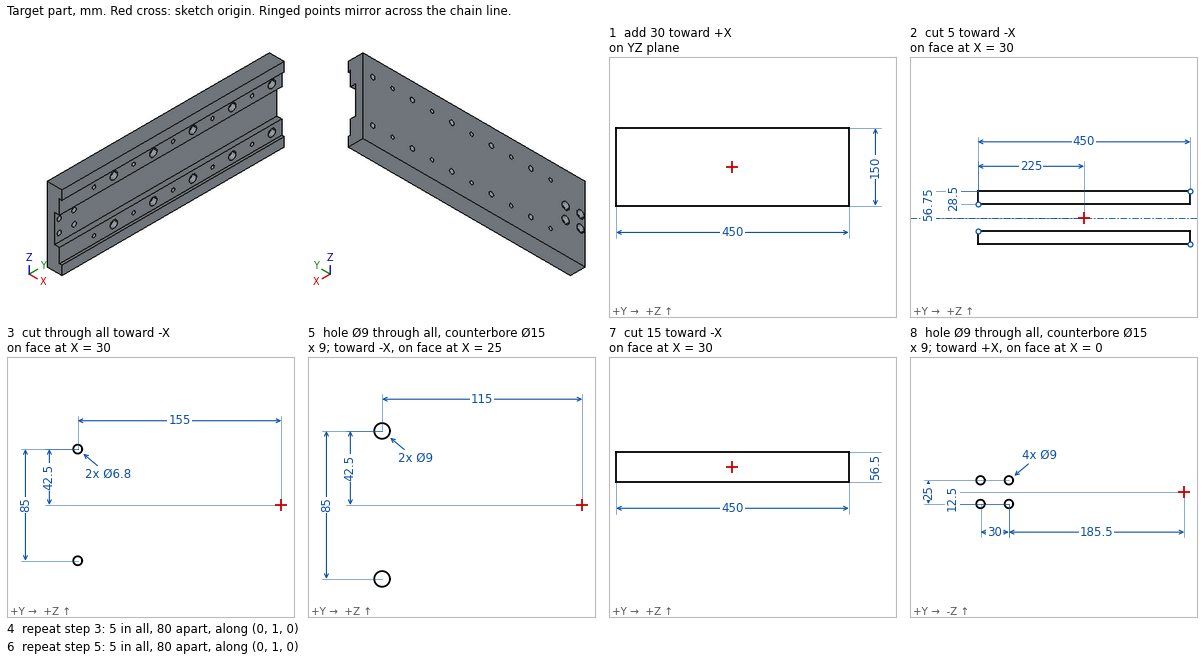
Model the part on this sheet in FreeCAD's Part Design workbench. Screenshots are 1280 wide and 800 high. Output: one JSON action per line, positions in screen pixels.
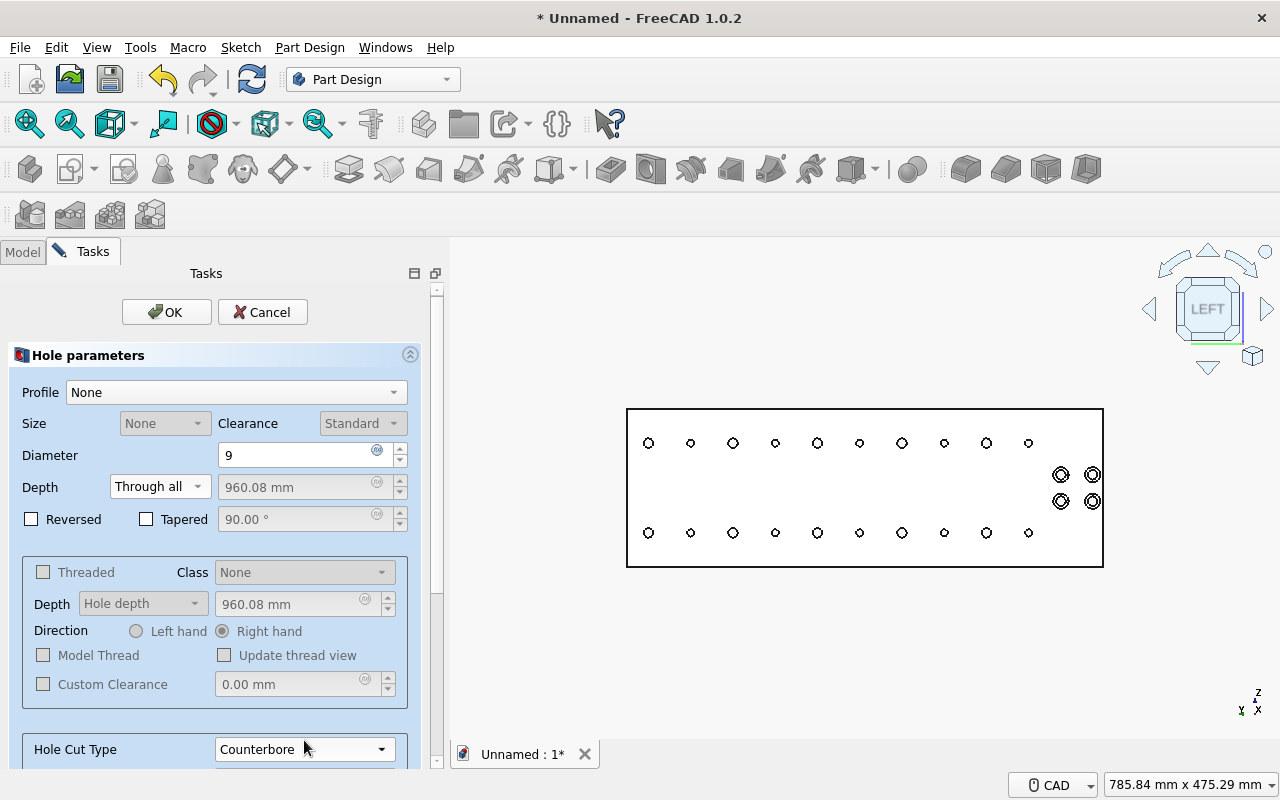
{"action": "scroll", "coordinate": [437, 526], "scroll_direction": "down", "scroll_amount": 2}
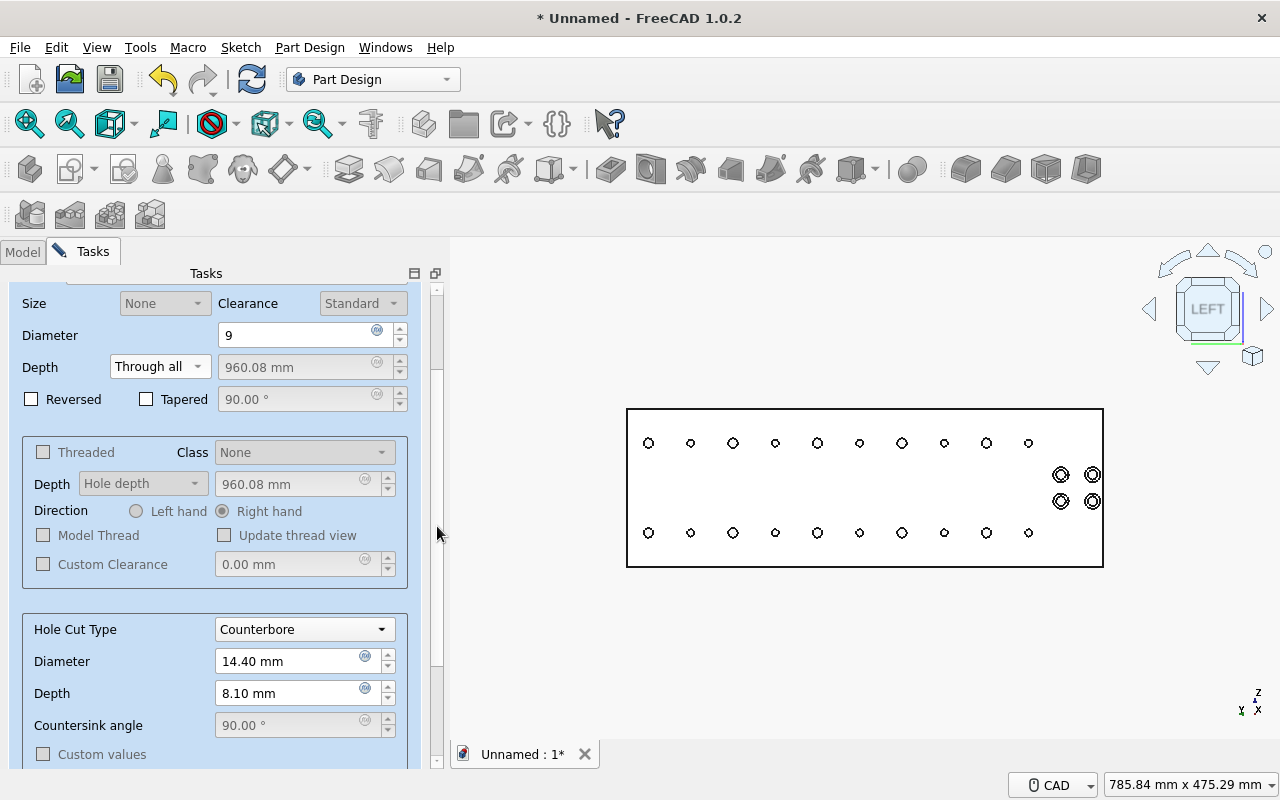
{"action": "triple_click", "coordinate": [298, 661]}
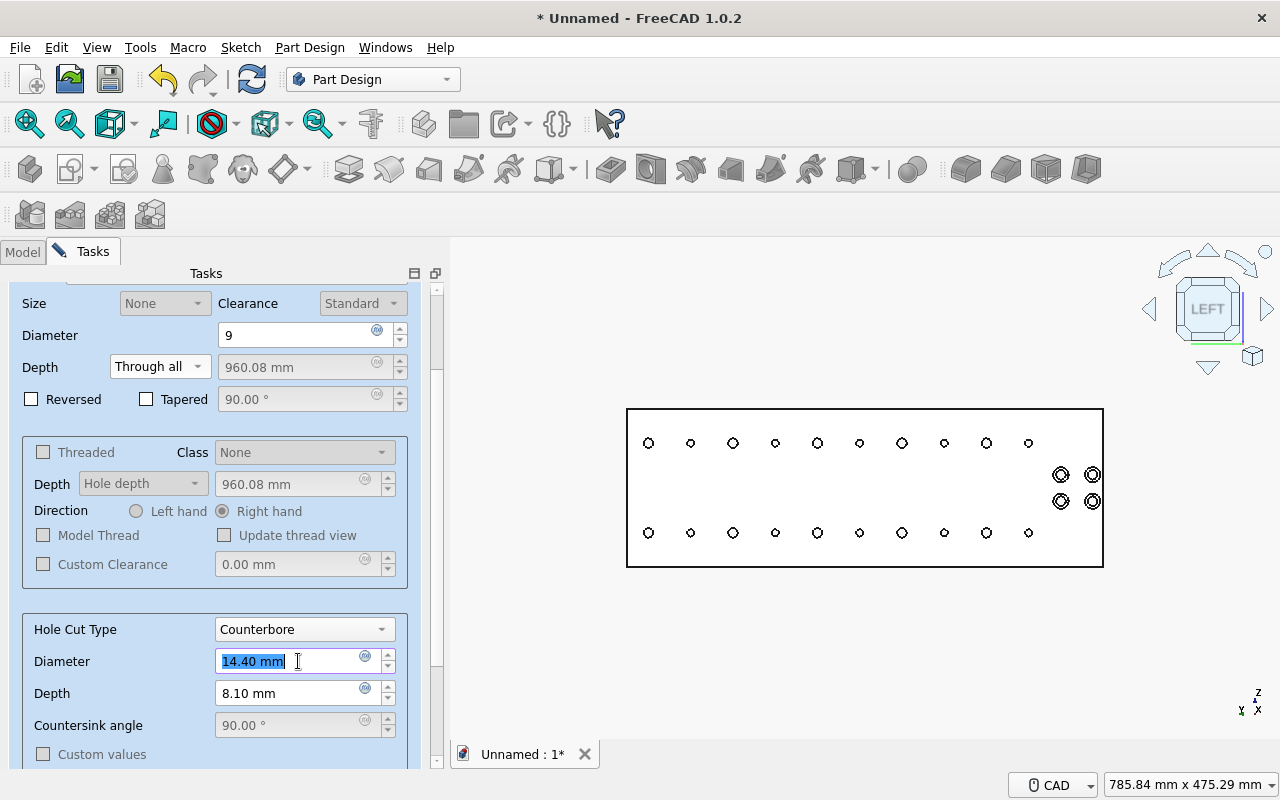
{"action": "type", "text": "15"}
{"action": "key", "text": "Tab"}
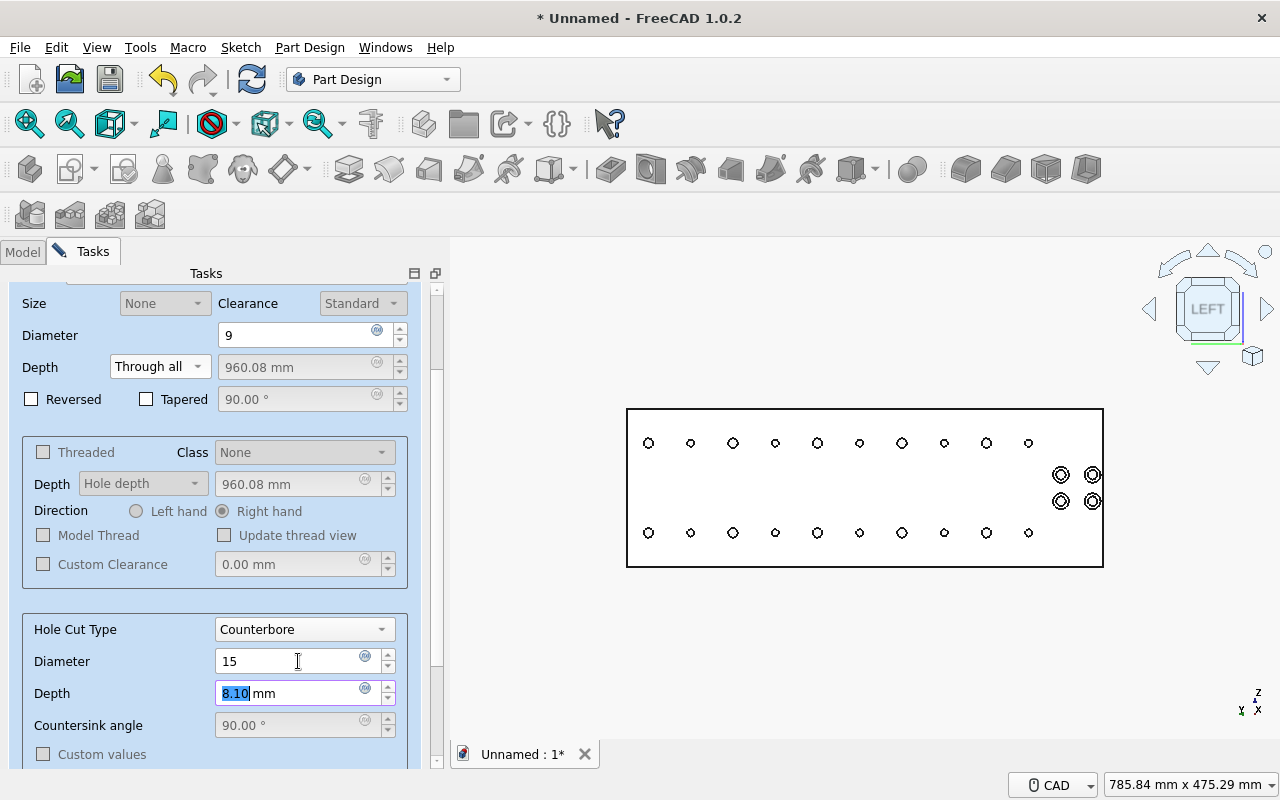
{"action": "type", "text": "9"}
{"action": "key", "text": "Tab"}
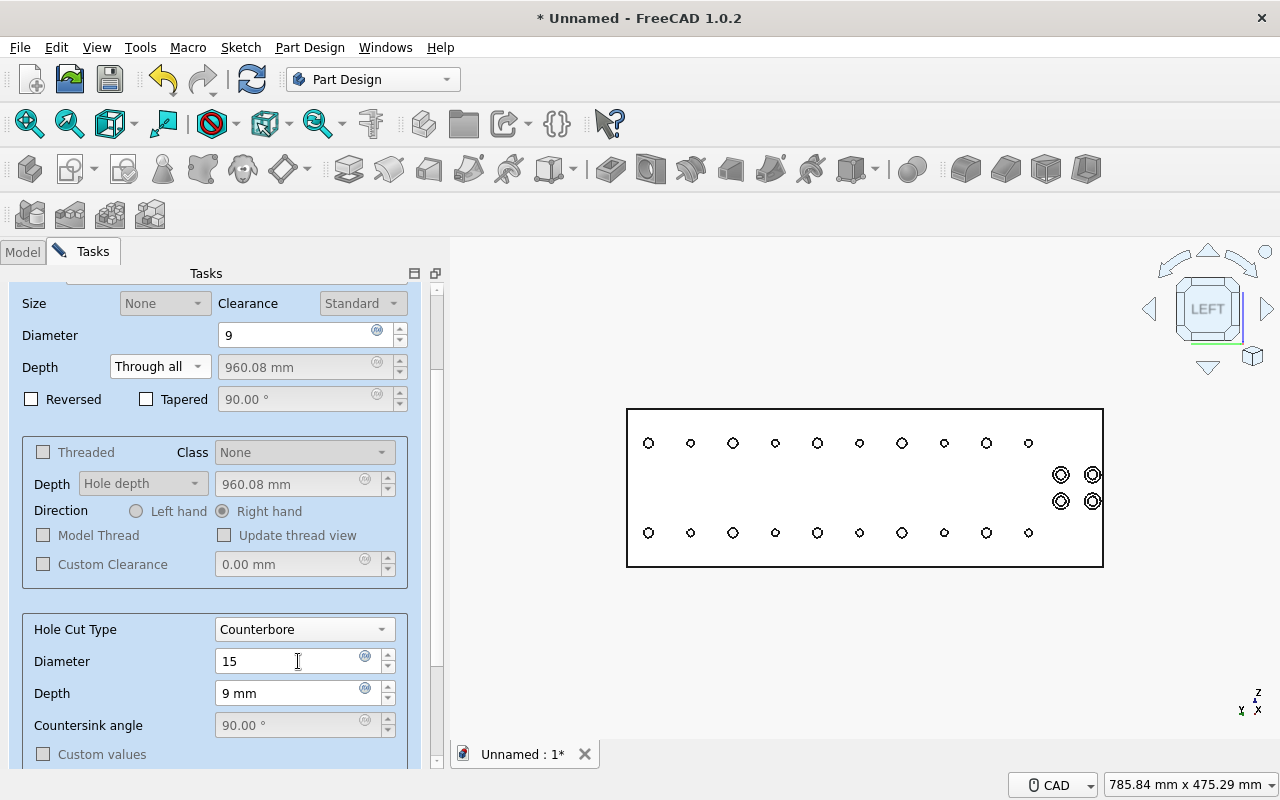
{"action": "scroll", "coordinate": [437, 526], "scroll_direction": "up", "scroll_amount": 3}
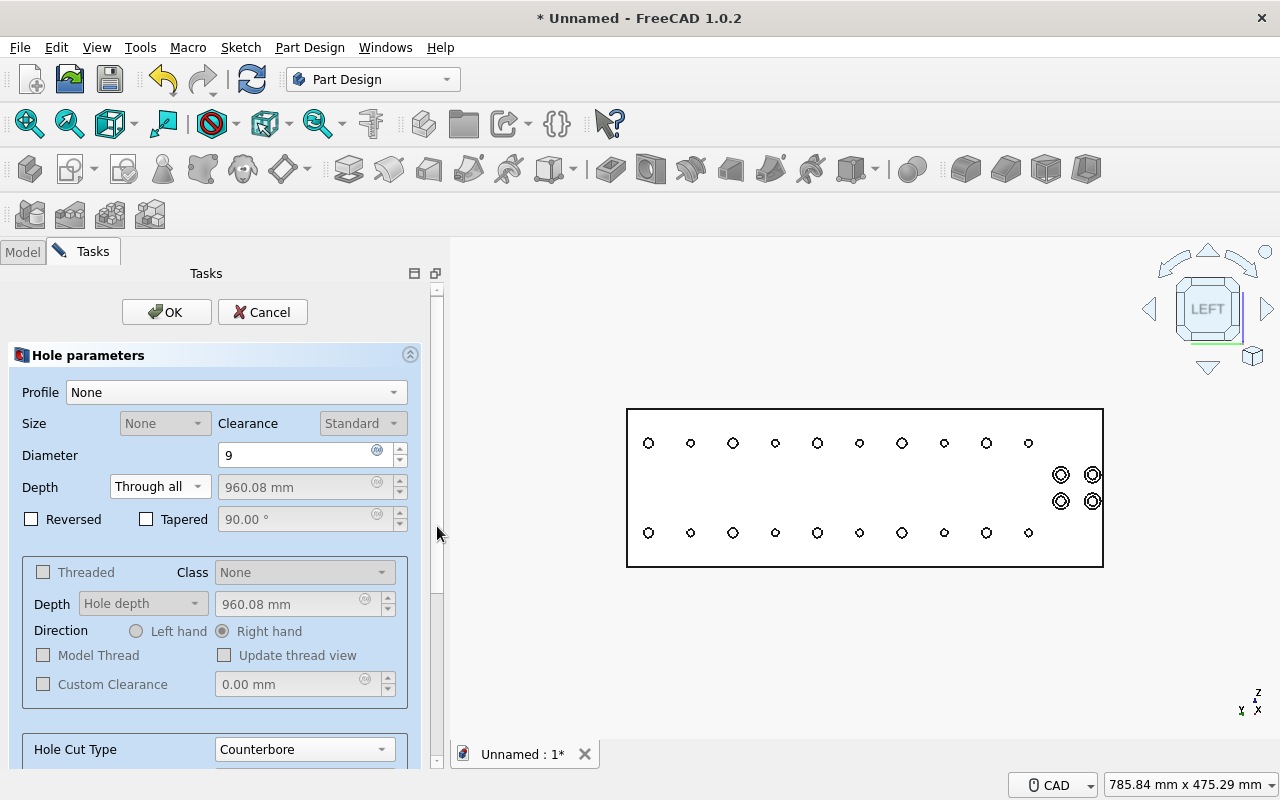
{"action": "left_click", "coordinate": [167, 312]}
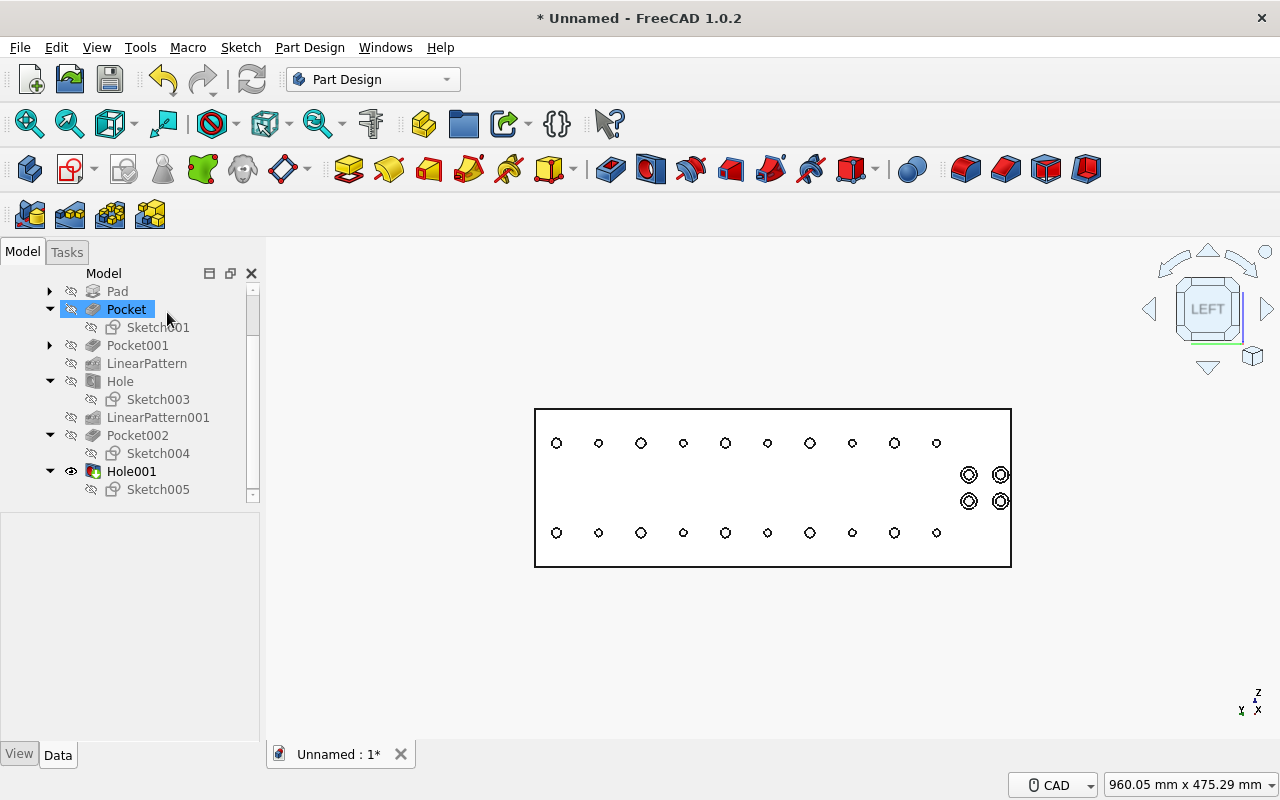
{"action": "key", "text": "0"}